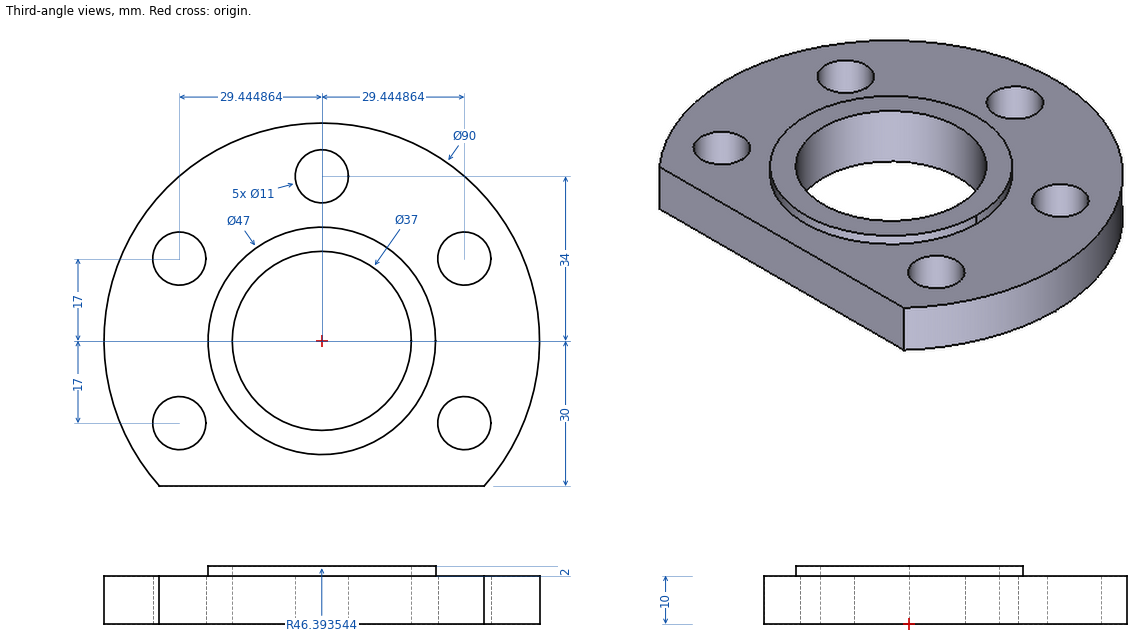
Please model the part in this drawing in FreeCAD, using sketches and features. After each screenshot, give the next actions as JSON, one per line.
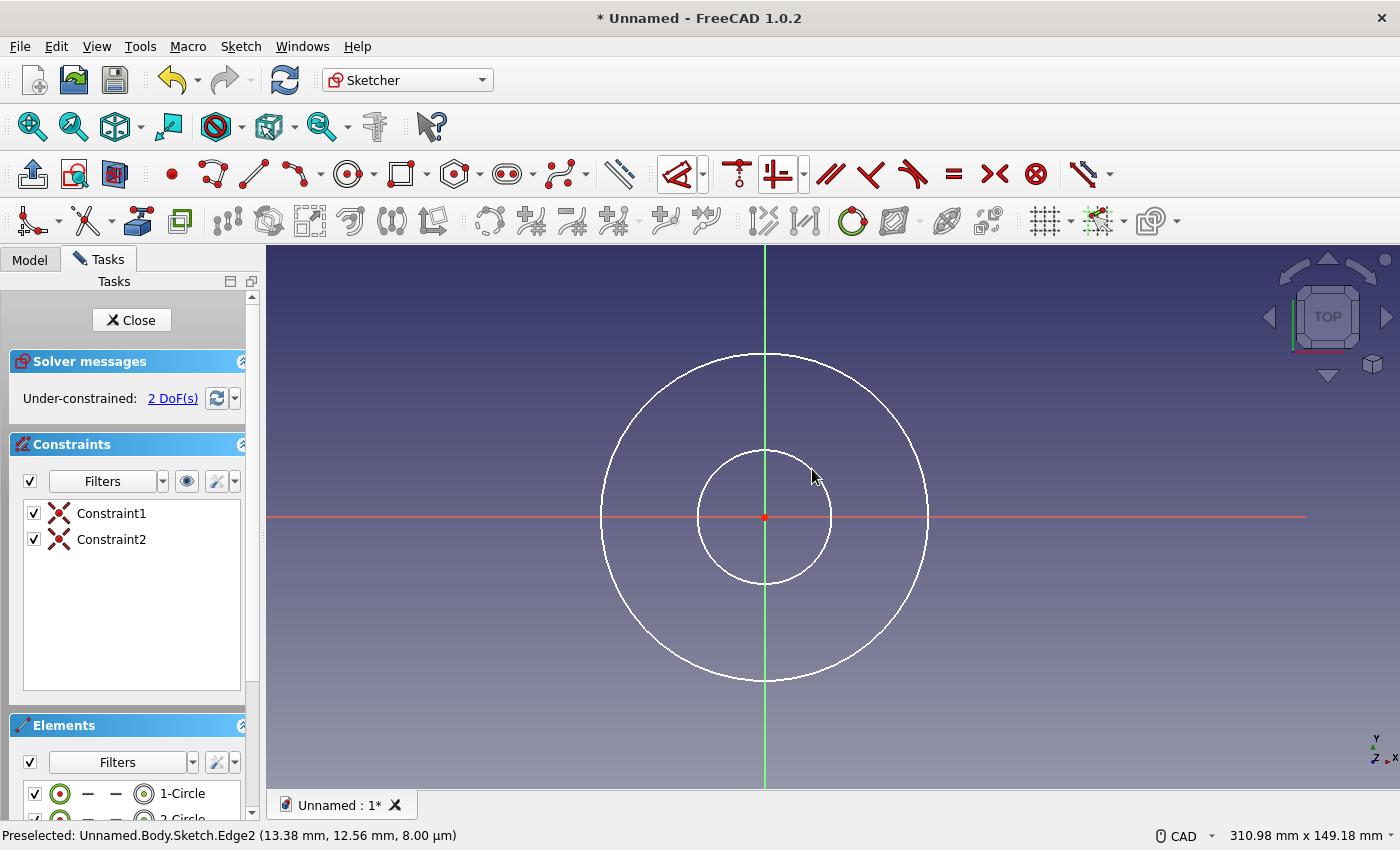
{"action": "left_click", "coordinate": [676, 174]}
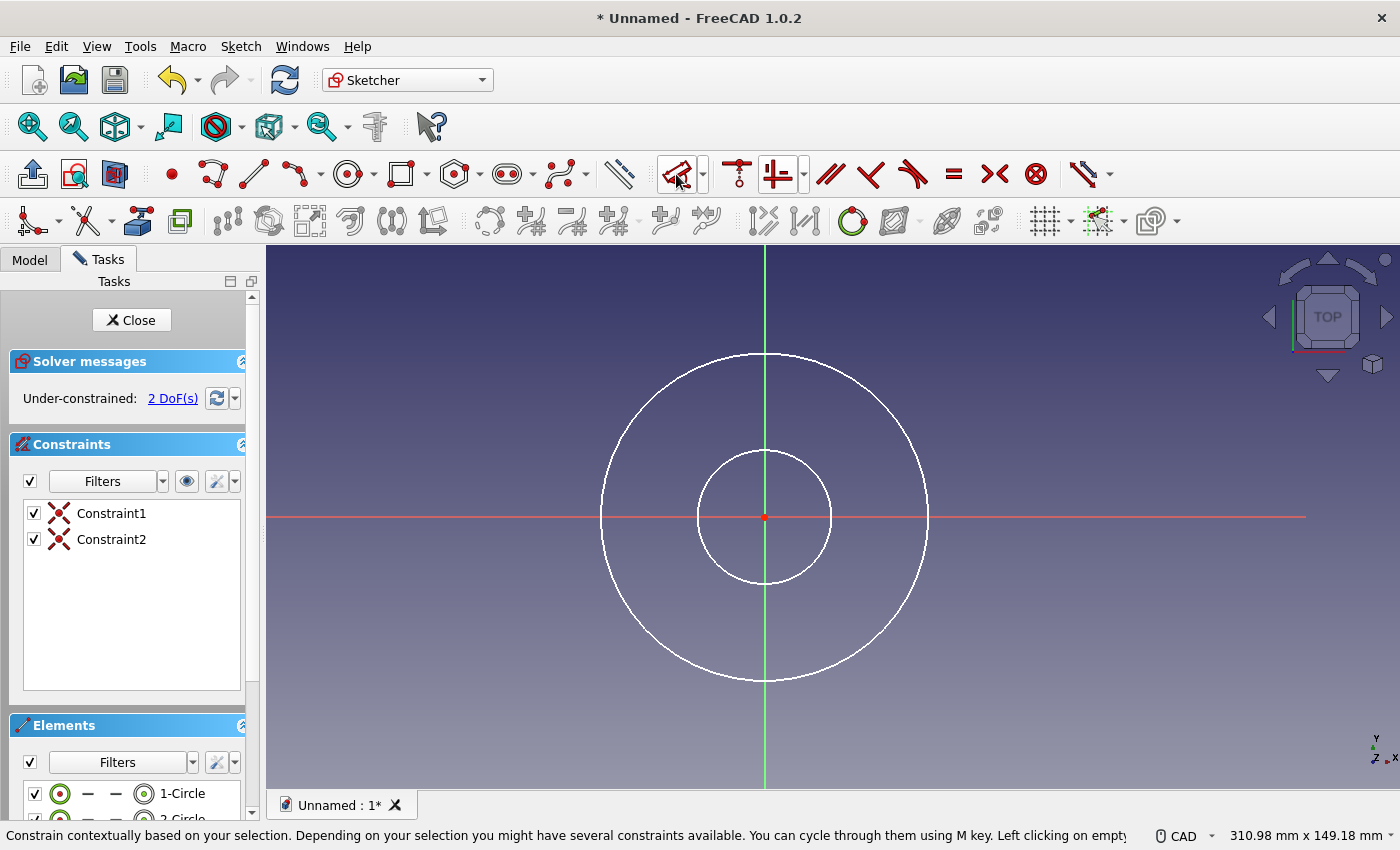
{"action": "left_click", "coordinate": [880, 401]}
{"action": "left_click", "coordinate": [903, 378]}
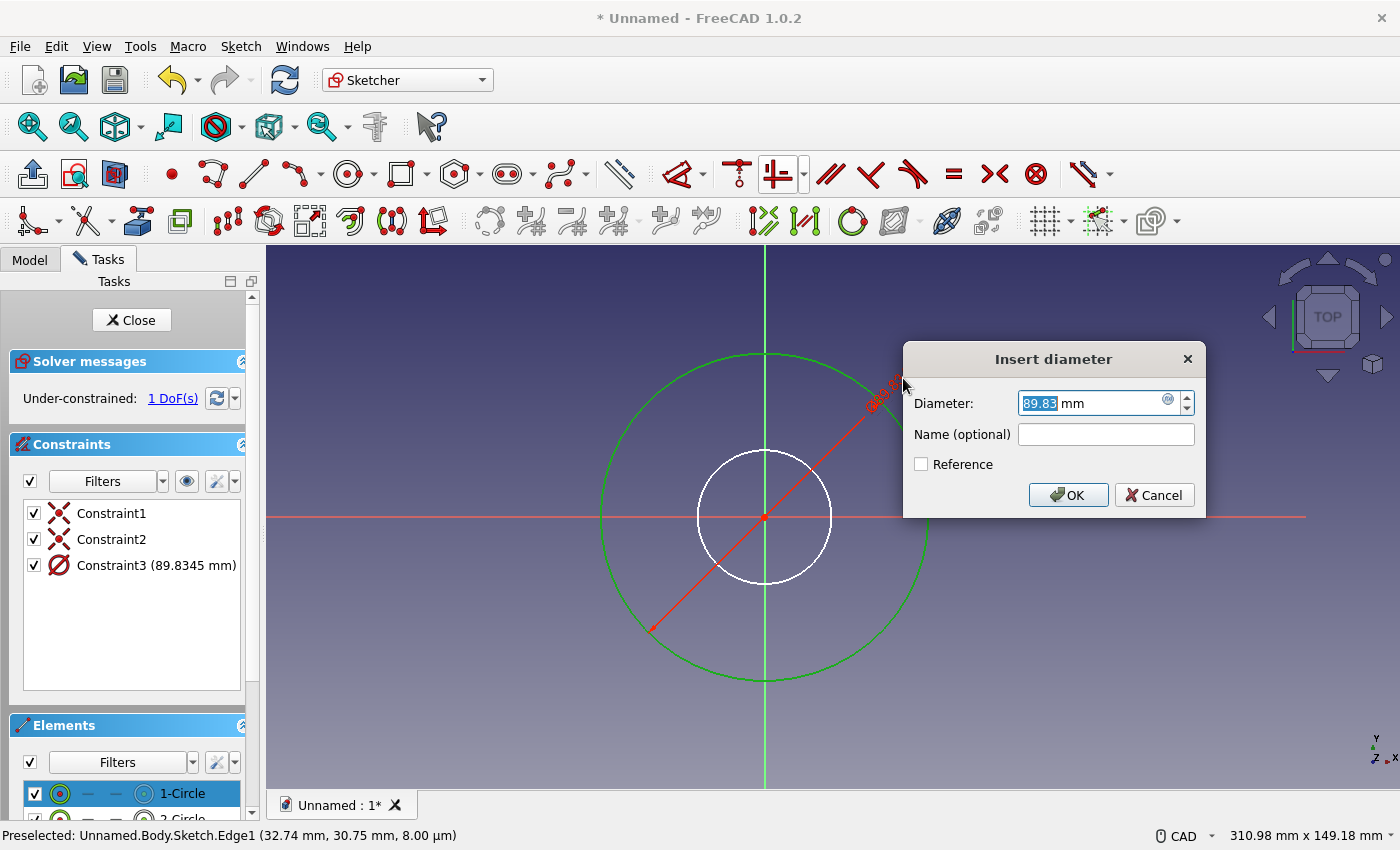
{"action": "type", "text": "90"}
{"action": "key", "text": "Return"}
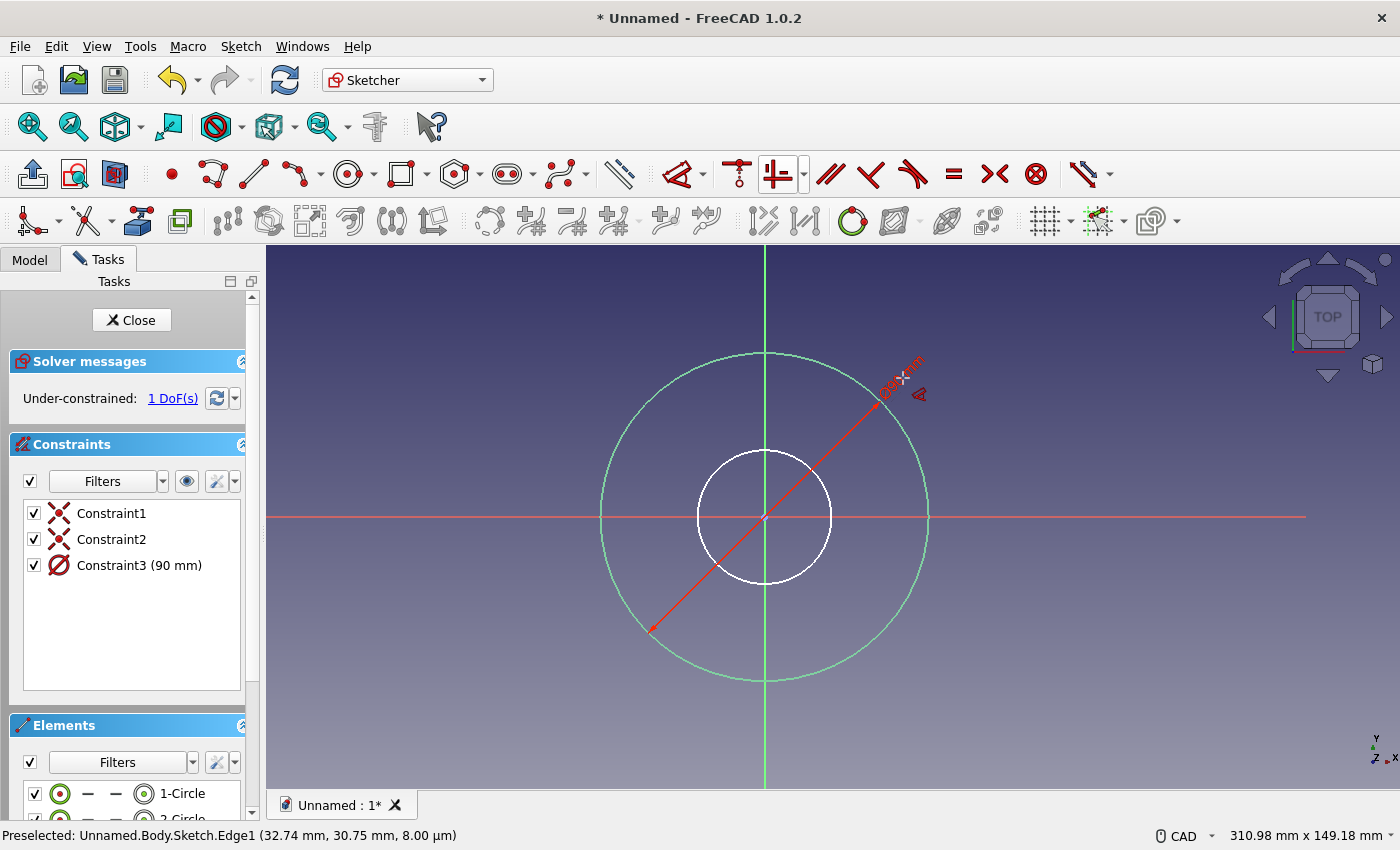
{"action": "left_click", "coordinate": [812, 470]}
{"action": "left_click", "coordinate": [835, 447]}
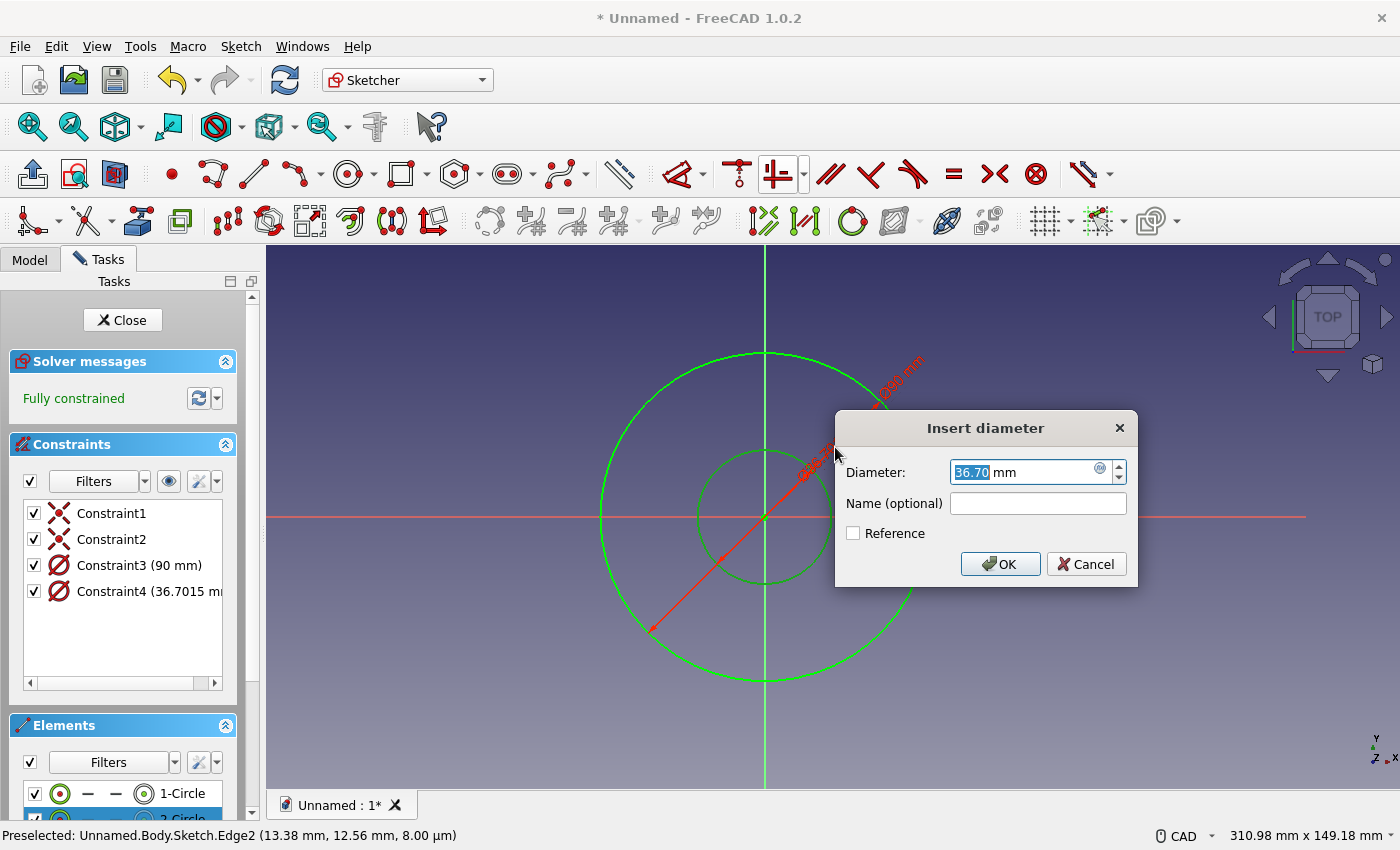
{"action": "type", "text": "37"}
{"action": "key", "text": "Return"}
{"action": "key", "text": "Escape"}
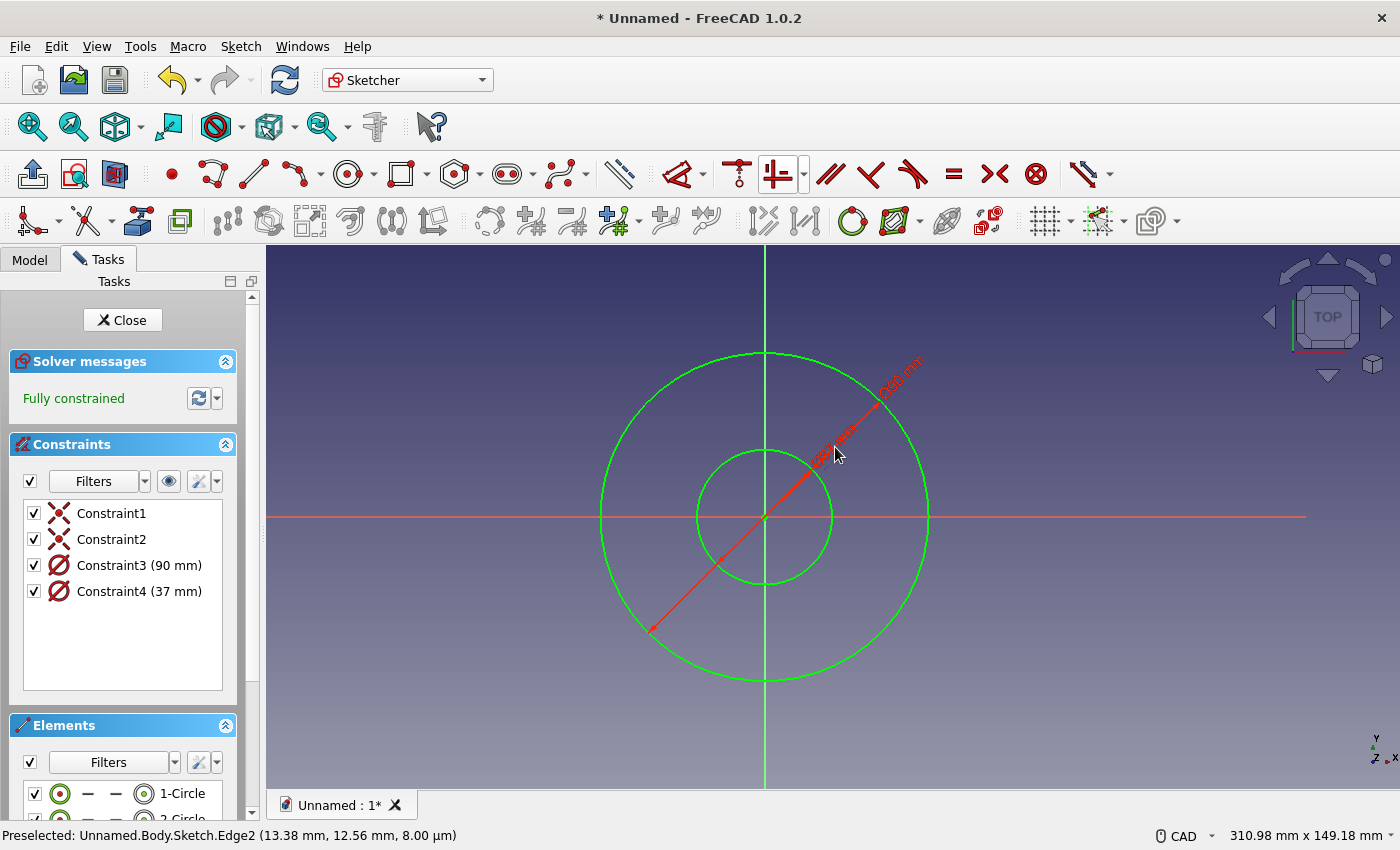
{"action": "left_click", "coordinate": [123, 320]}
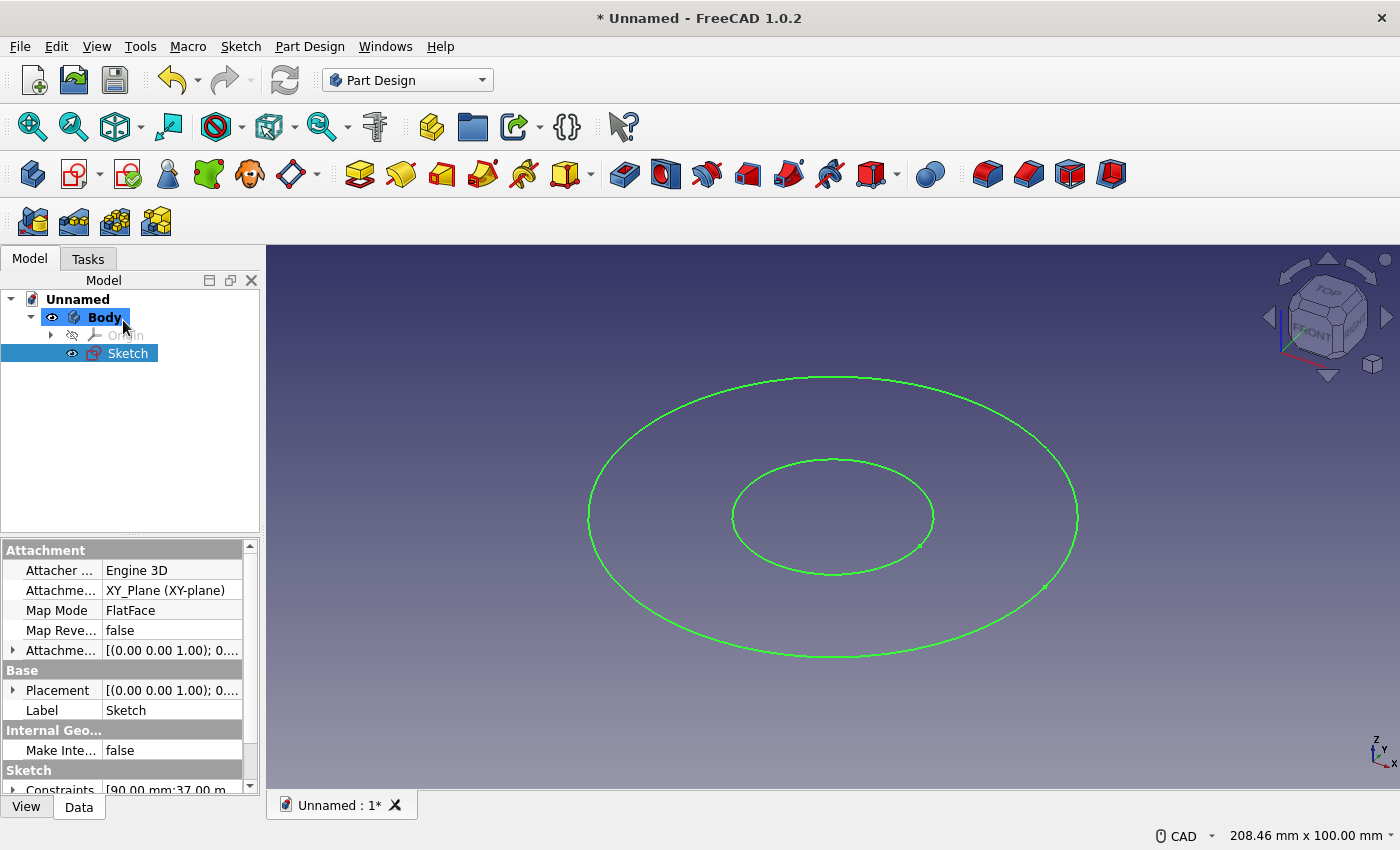
{"action": "left_click", "coordinate": [360, 174]}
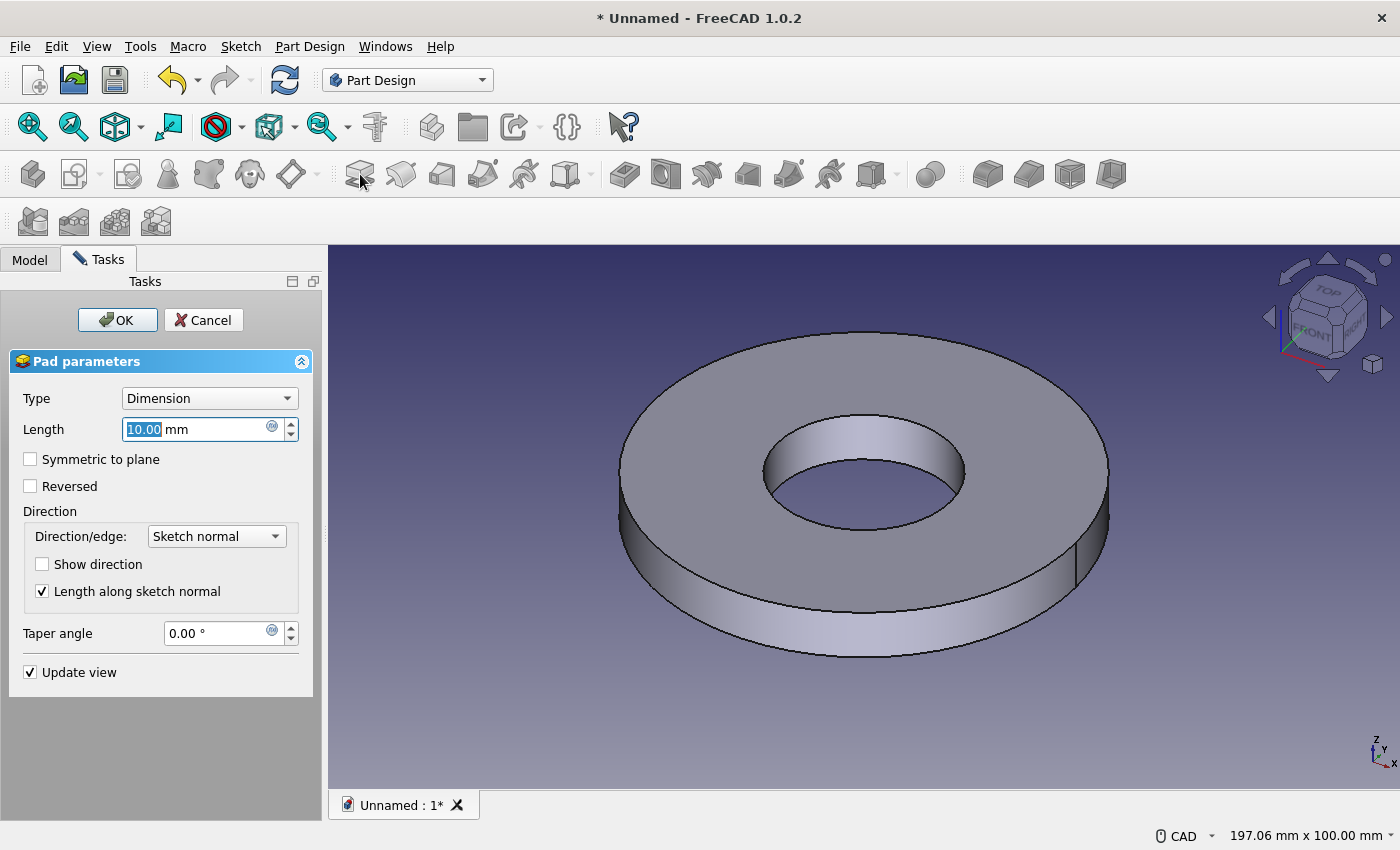
{"action": "type", "text": "10"}
{"action": "key", "text": "Tab"}